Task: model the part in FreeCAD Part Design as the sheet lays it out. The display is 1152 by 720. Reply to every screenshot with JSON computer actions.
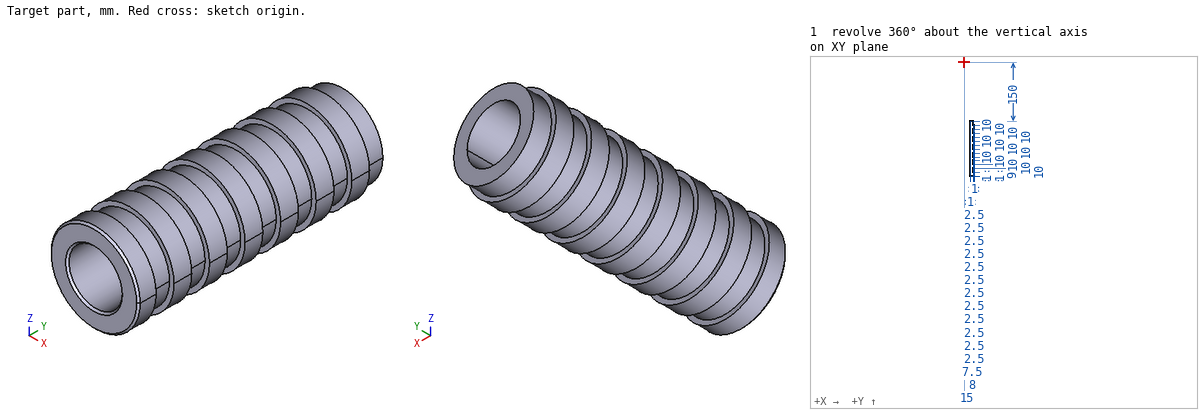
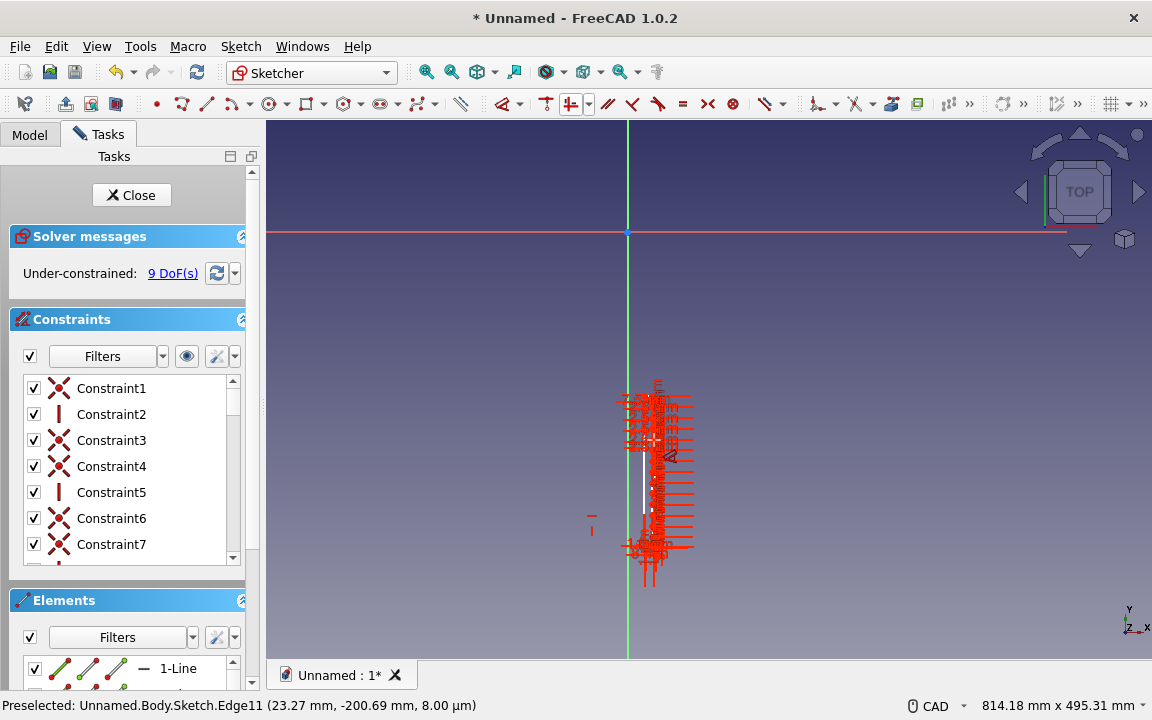
{"action": "scroll", "coordinate": [654, 461], "scroll_direction": "up", "scroll_amount": 14}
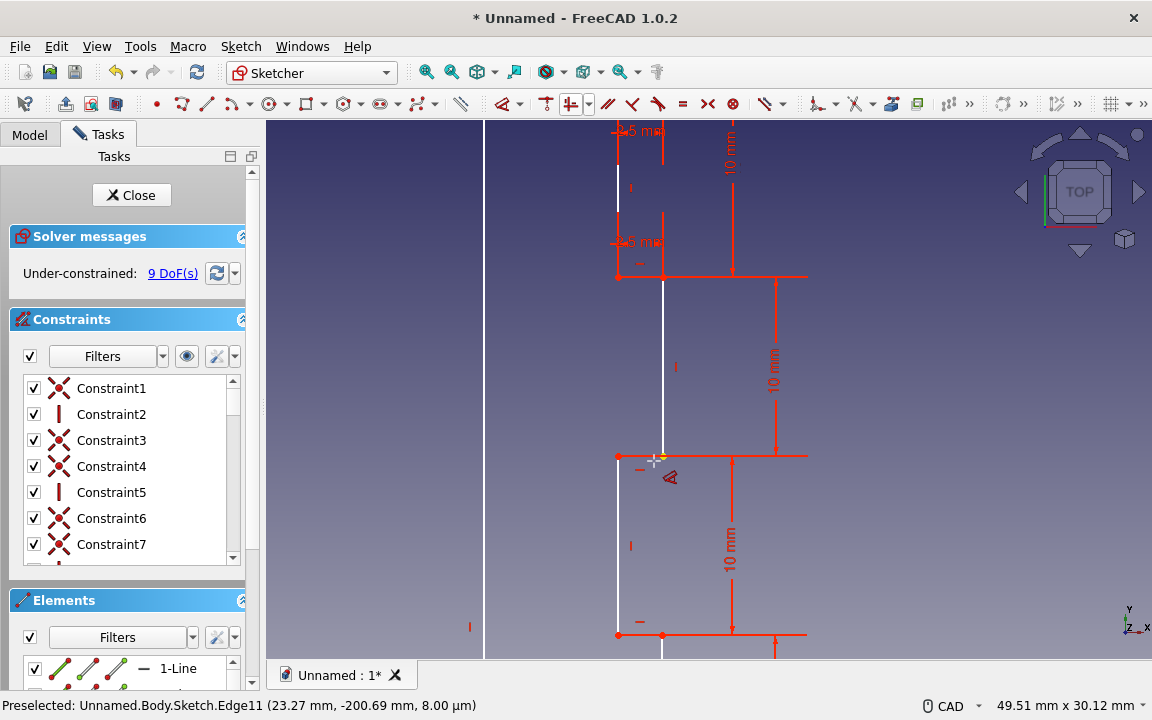
{"action": "left_click", "coordinate": [650, 456]}
{"action": "left_click", "coordinate": [641, 490]}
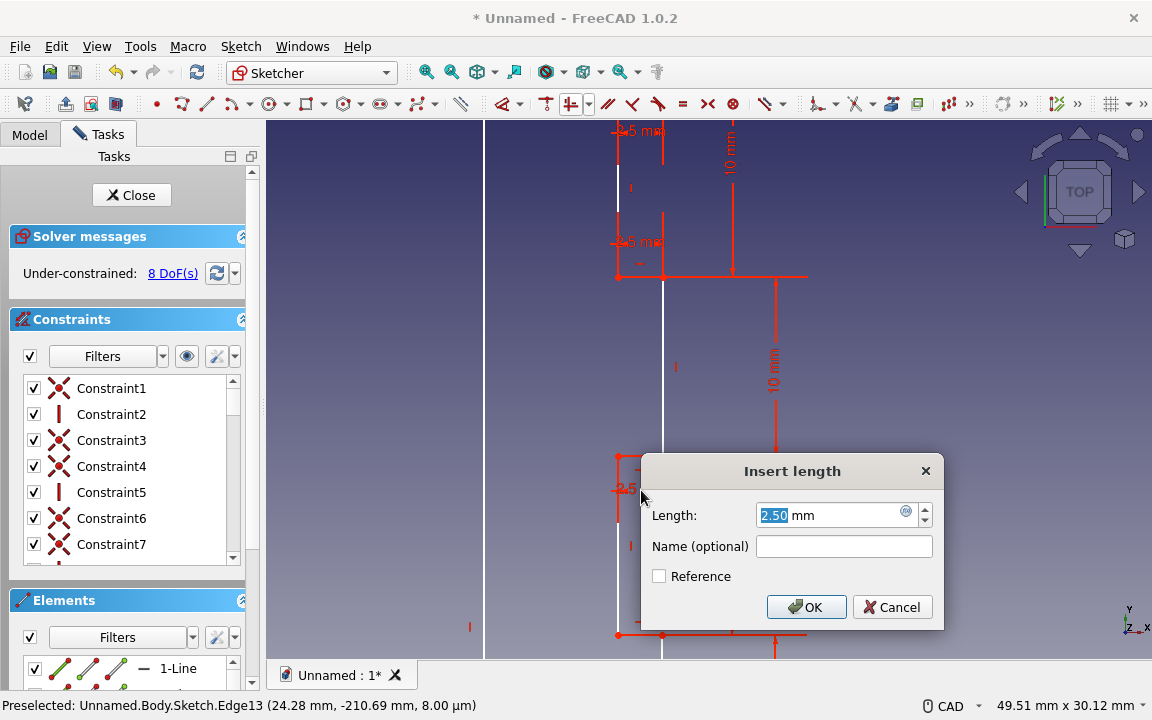
{"action": "type", "text": "2.5"}
{"action": "key", "text": "Return"}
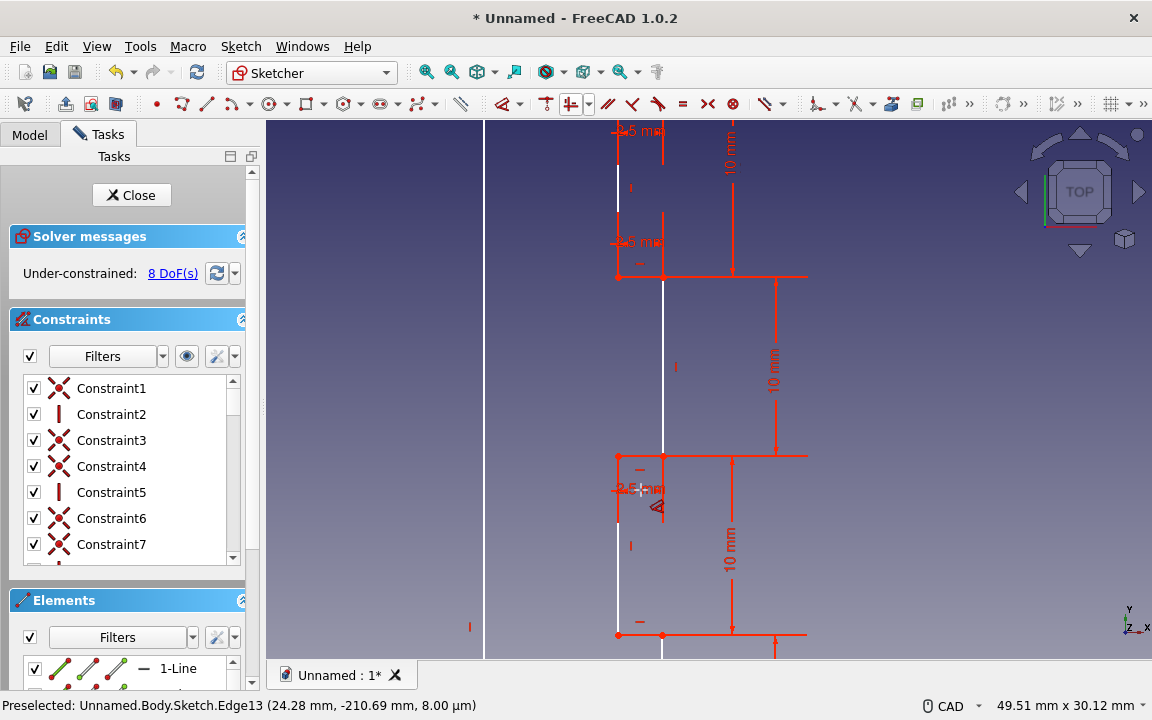
{"action": "scroll", "coordinate": [654, 461], "scroll_direction": "down", "scroll_amount": 14}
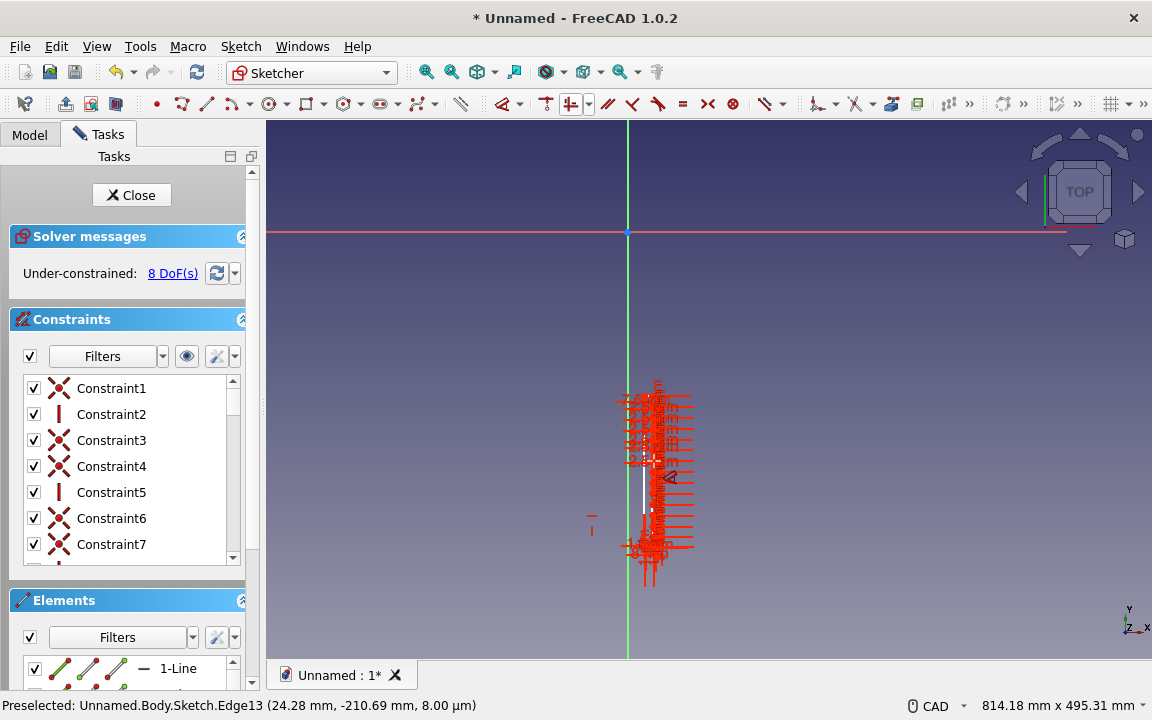
{"action": "scroll", "coordinate": [653, 472], "scroll_direction": "up", "scroll_amount": 14}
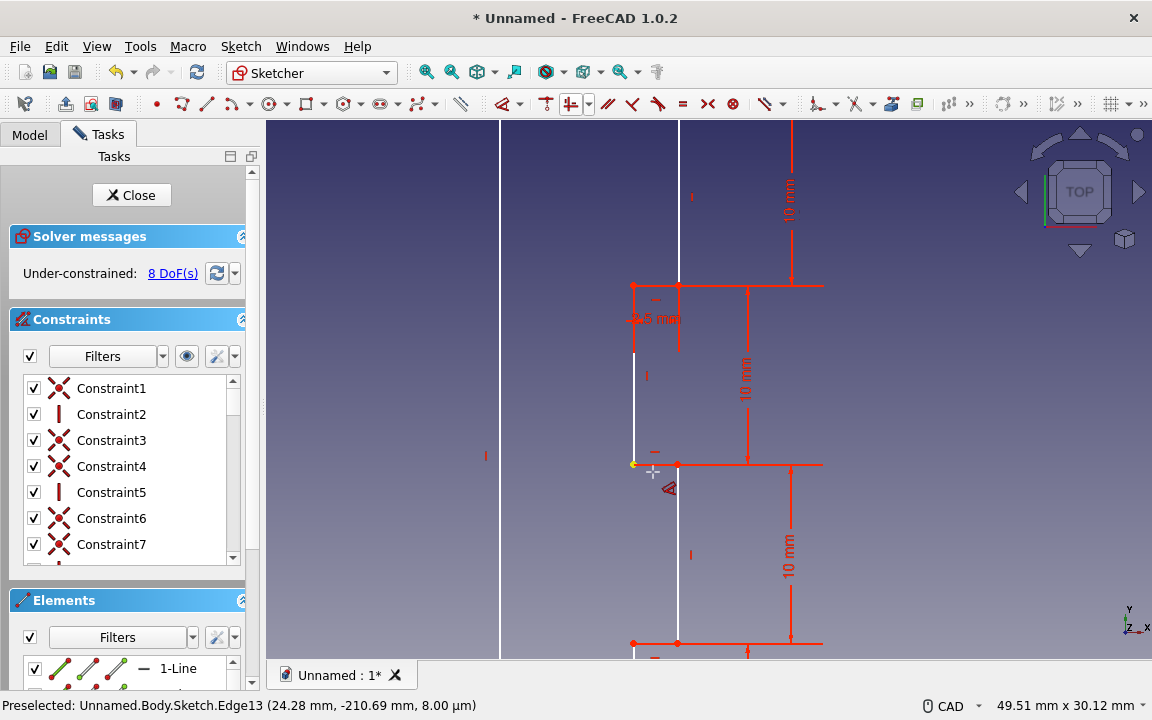
{"action": "left_click", "coordinate": [647, 465]}
{"action": "left_click", "coordinate": [656, 499]}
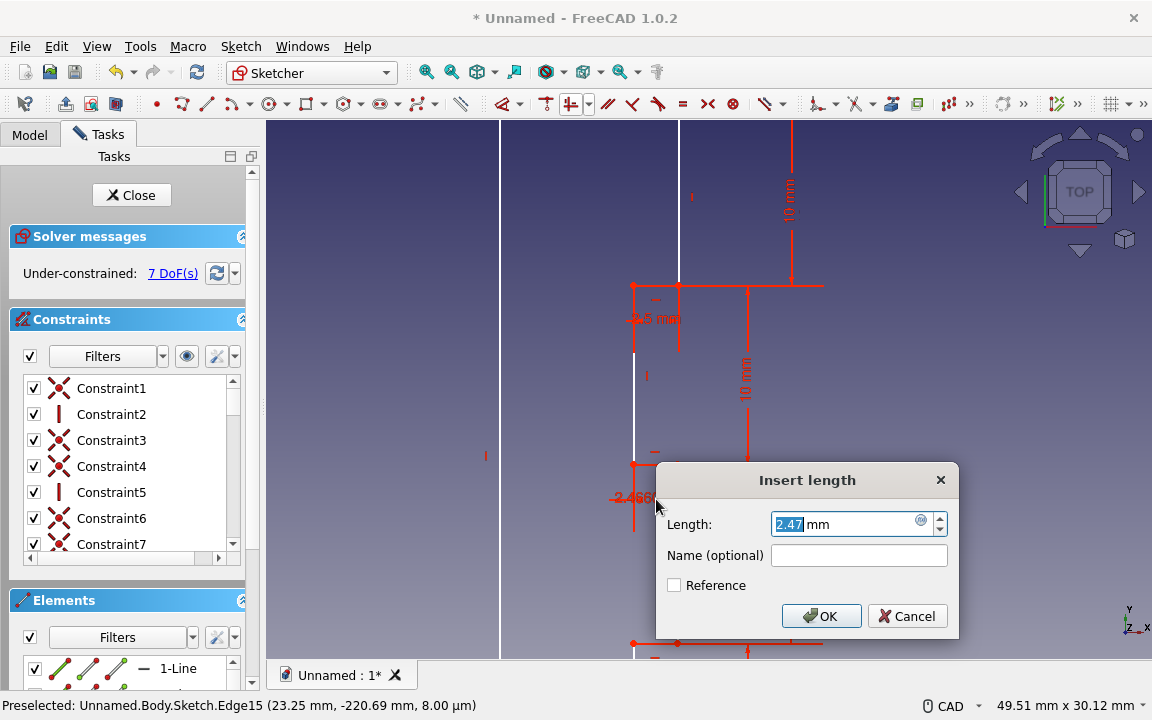
{"action": "type", "text": "2.5"}
{"action": "key", "text": "Return"}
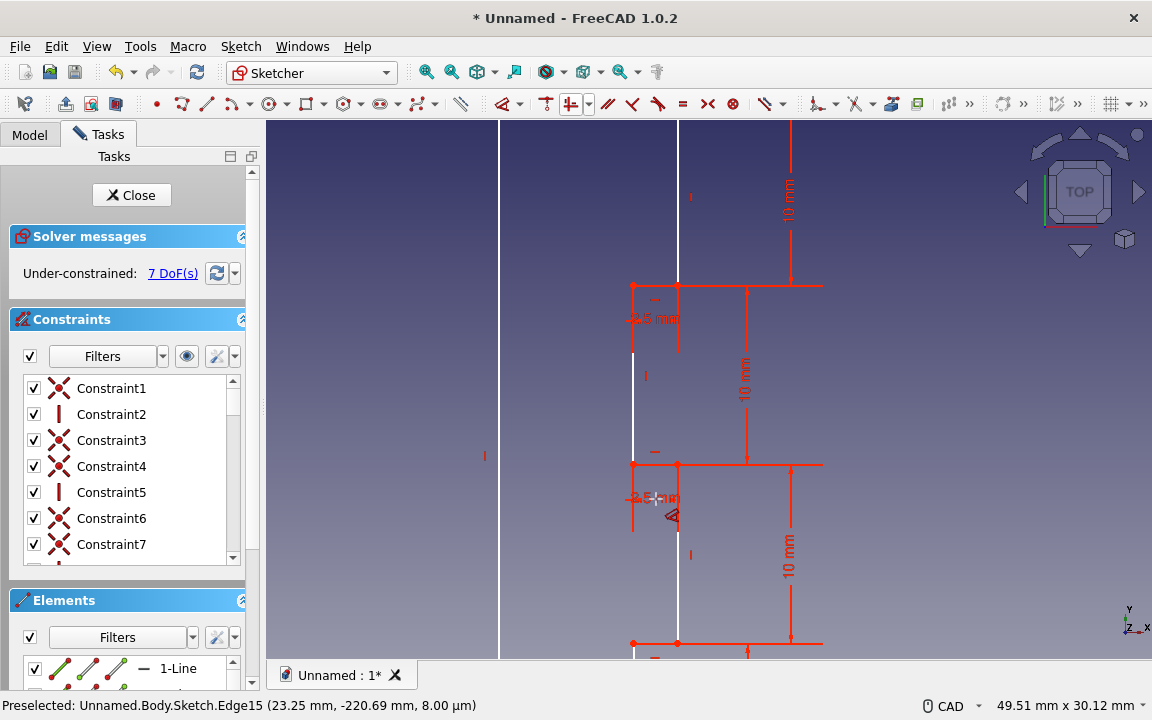
{"action": "scroll", "coordinate": [653, 472], "scroll_direction": "down", "scroll_amount": 14}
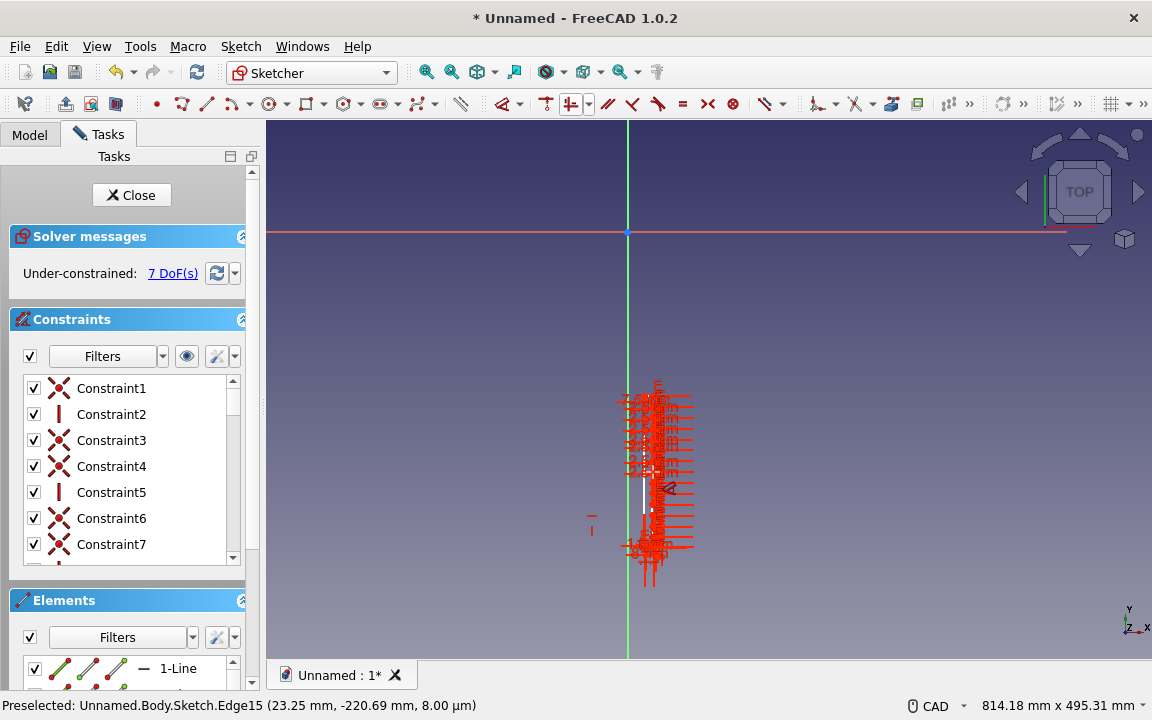
{"action": "scroll", "coordinate": [654, 483], "scroll_direction": "up", "scroll_amount": 14}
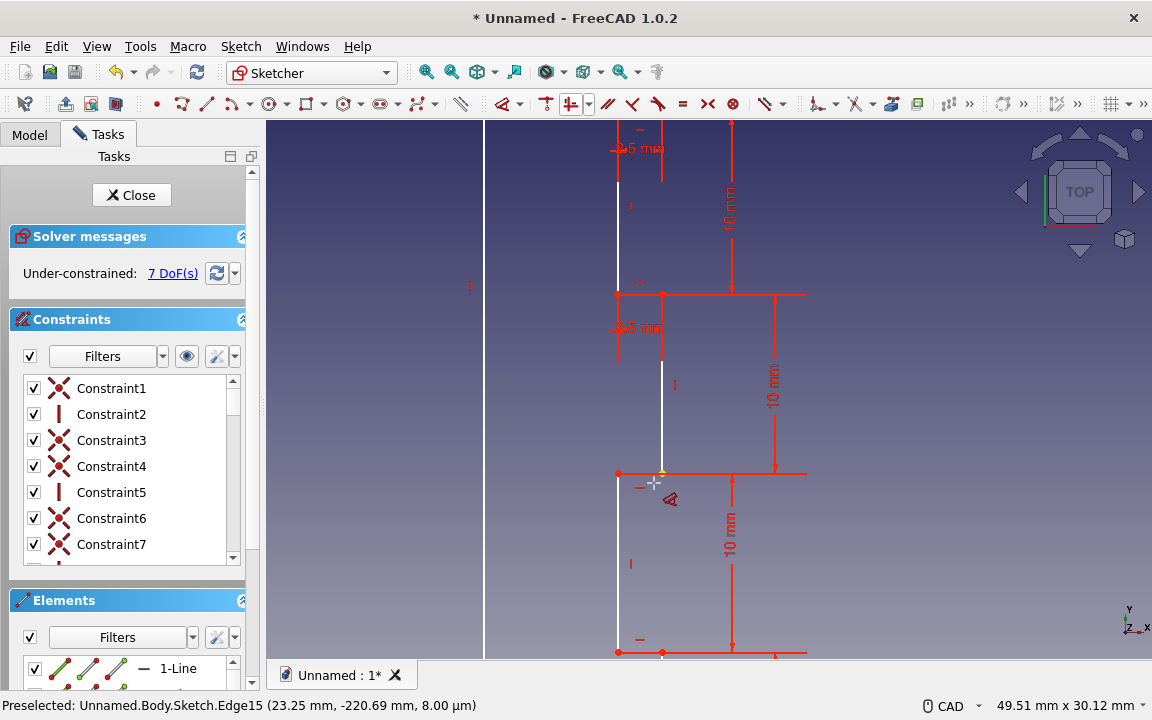
{"action": "left_click", "coordinate": [649, 474]}
{"action": "left_click", "coordinate": [640, 508]}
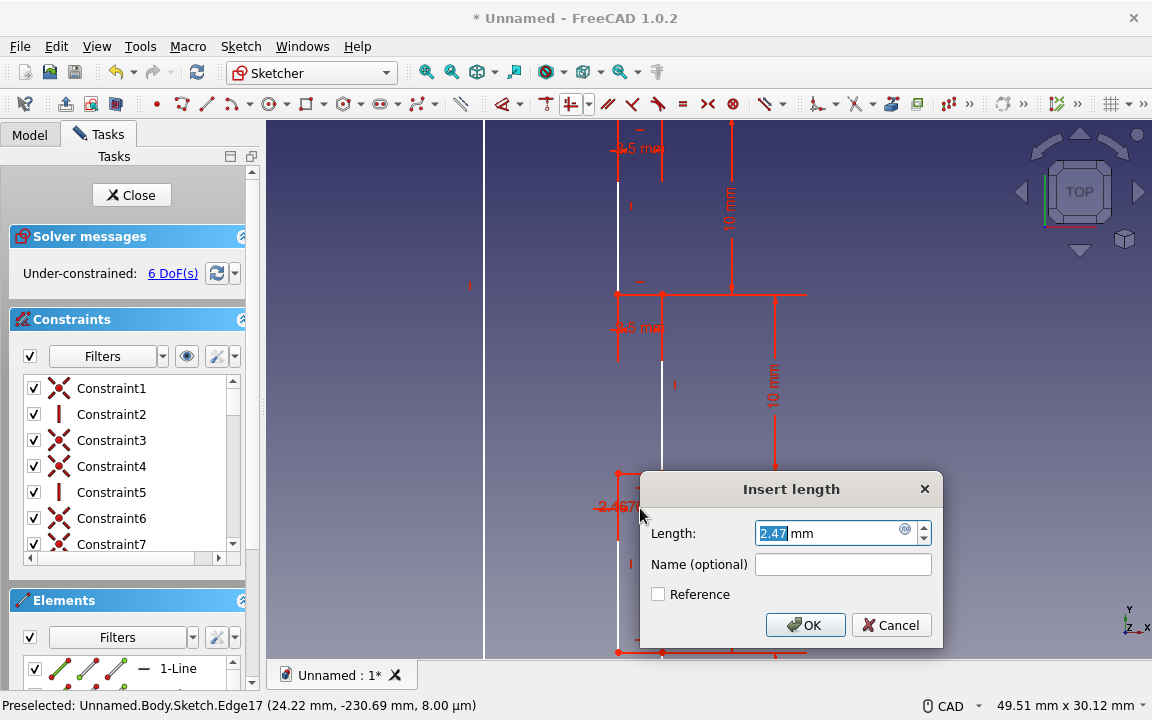
{"action": "type", "text": "2.5"}
{"action": "key", "text": "Return"}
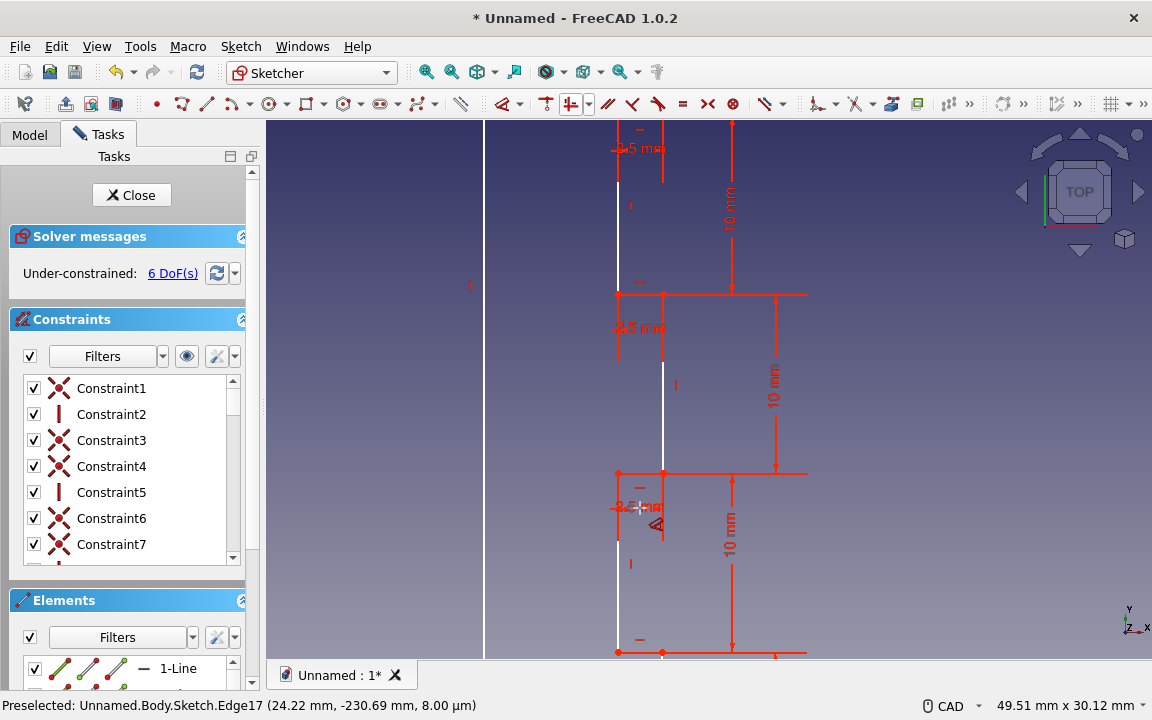
{"action": "scroll", "coordinate": [654, 483], "scroll_direction": "down", "scroll_amount": 14}